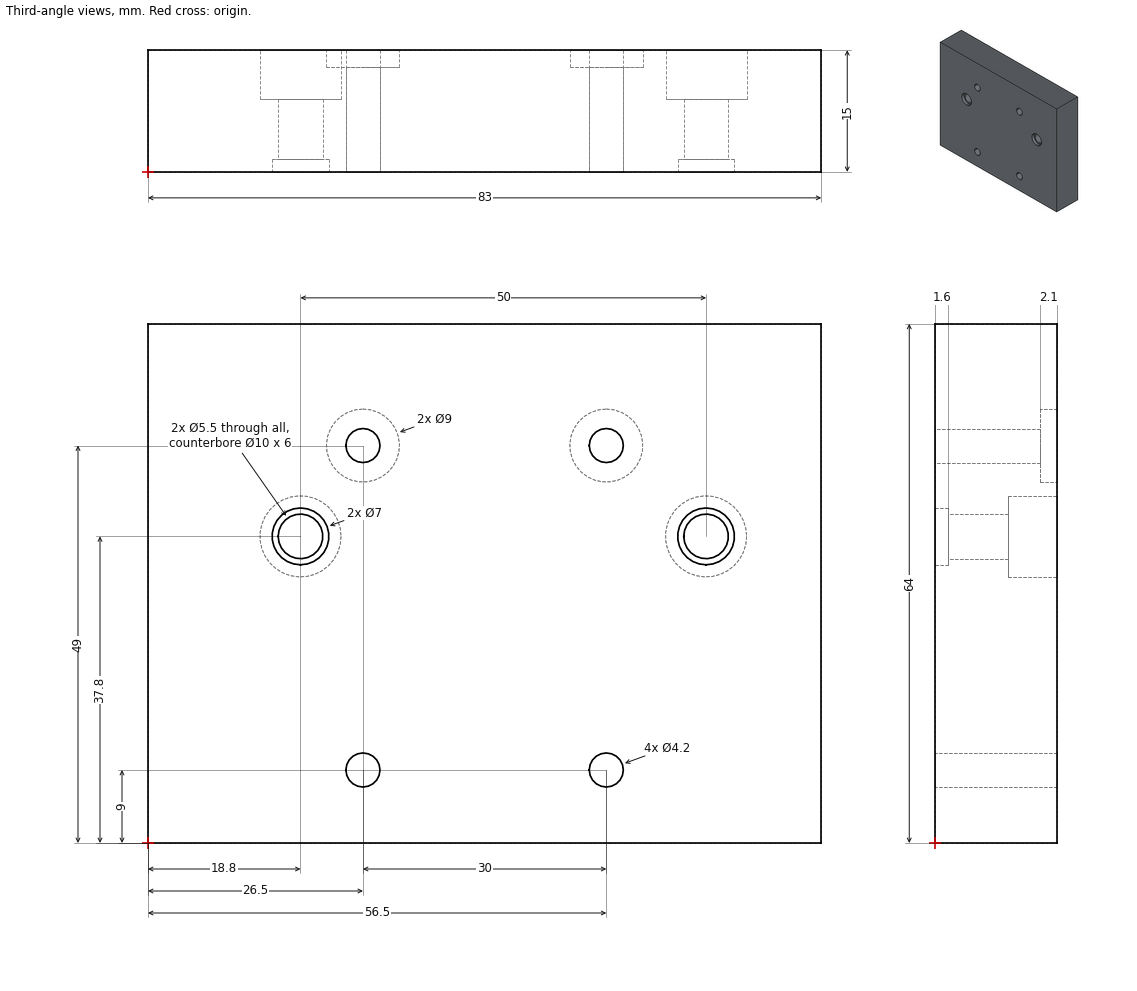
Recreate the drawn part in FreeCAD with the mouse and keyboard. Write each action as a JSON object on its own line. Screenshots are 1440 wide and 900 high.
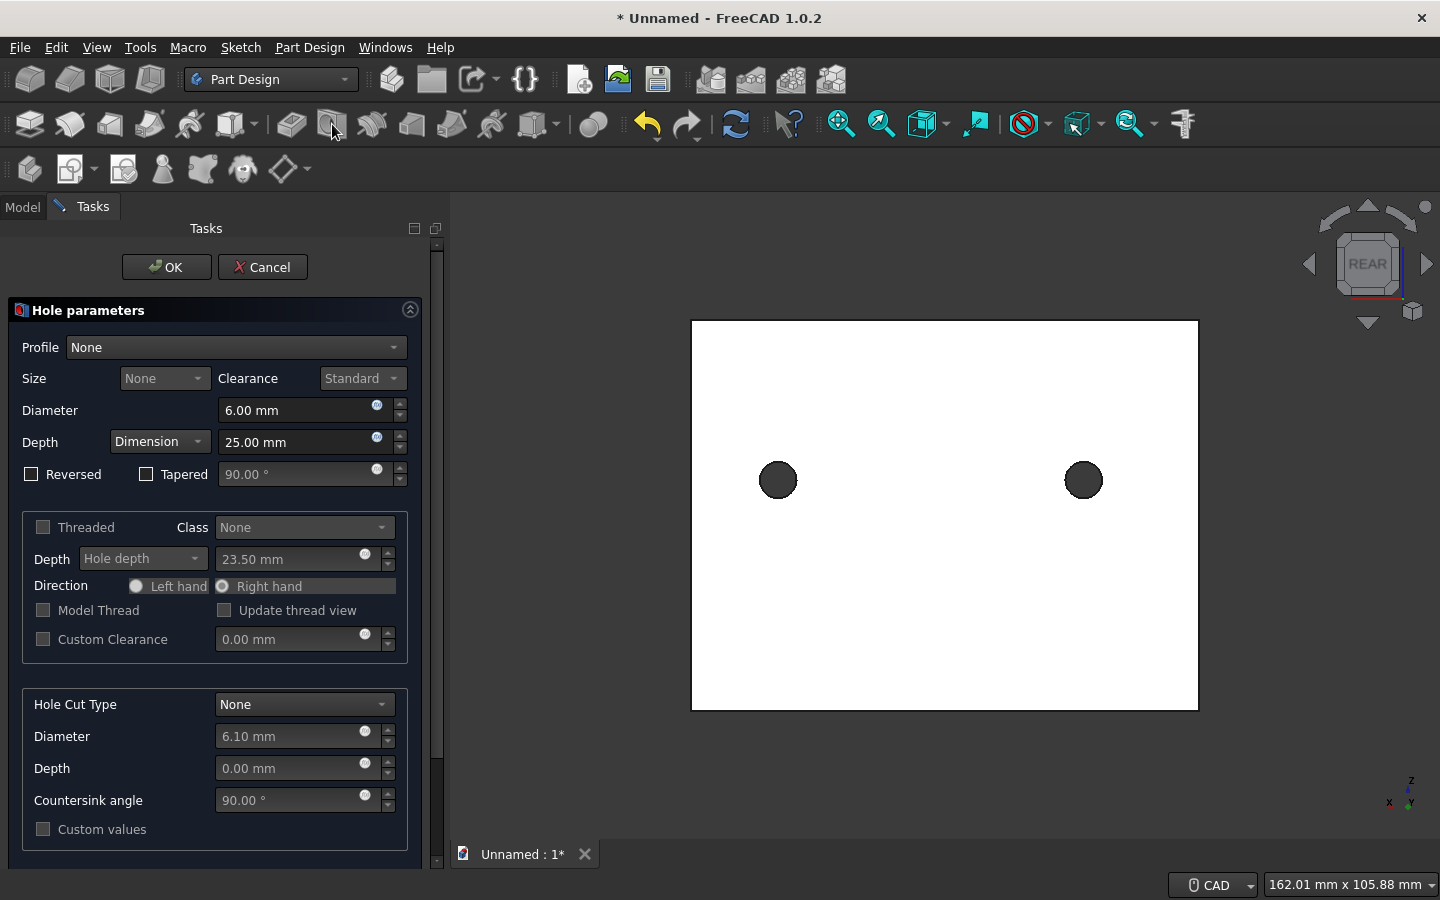
{"action": "triple_click", "coordinate": [305, 410]}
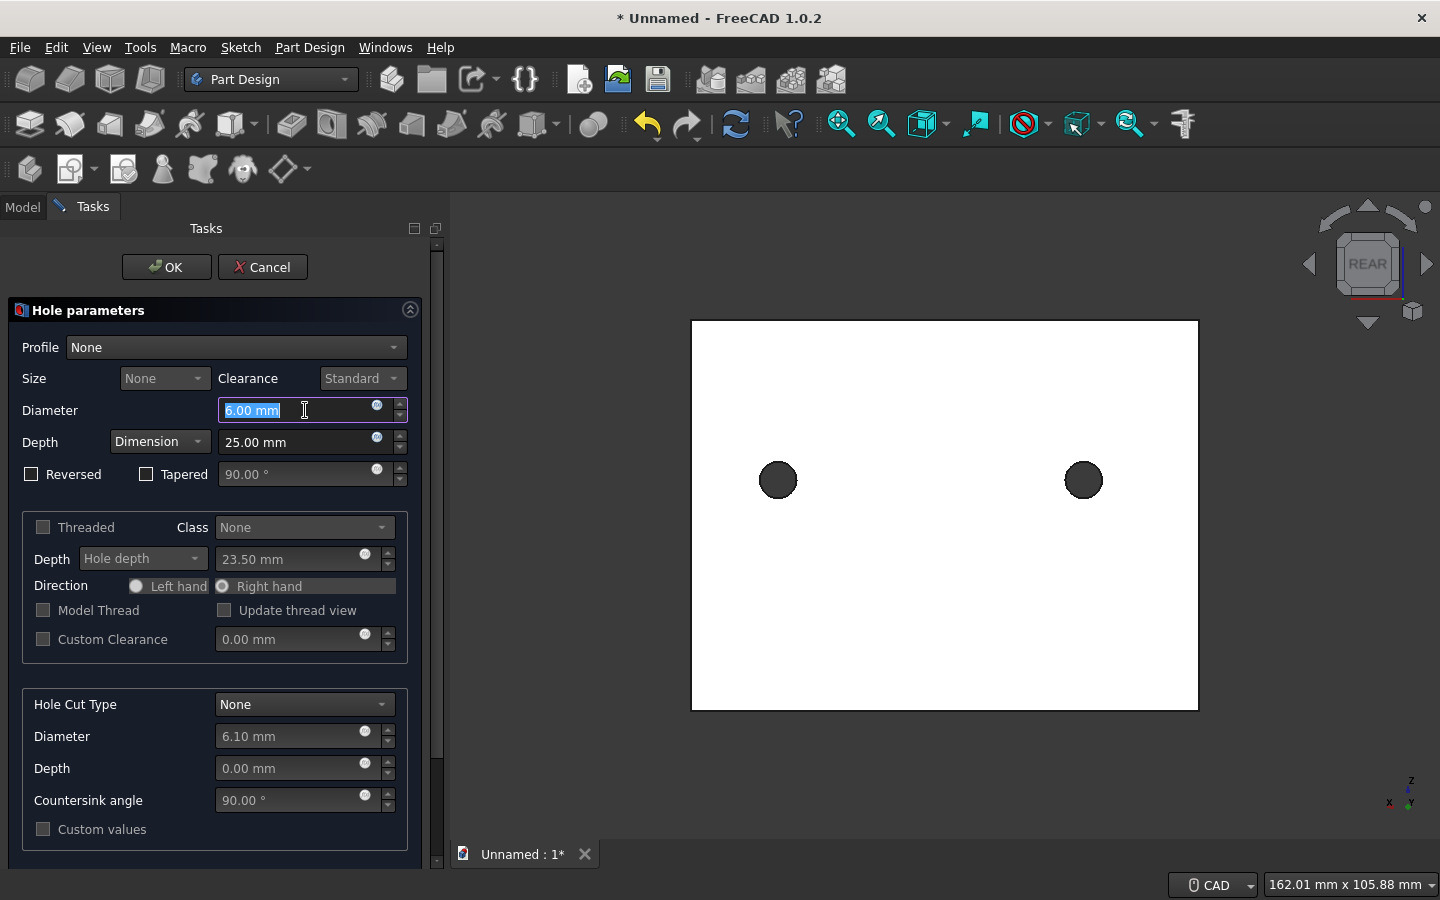
{"action": "type", "text": "5.5"}
{"action": "key", "text": "Tab"}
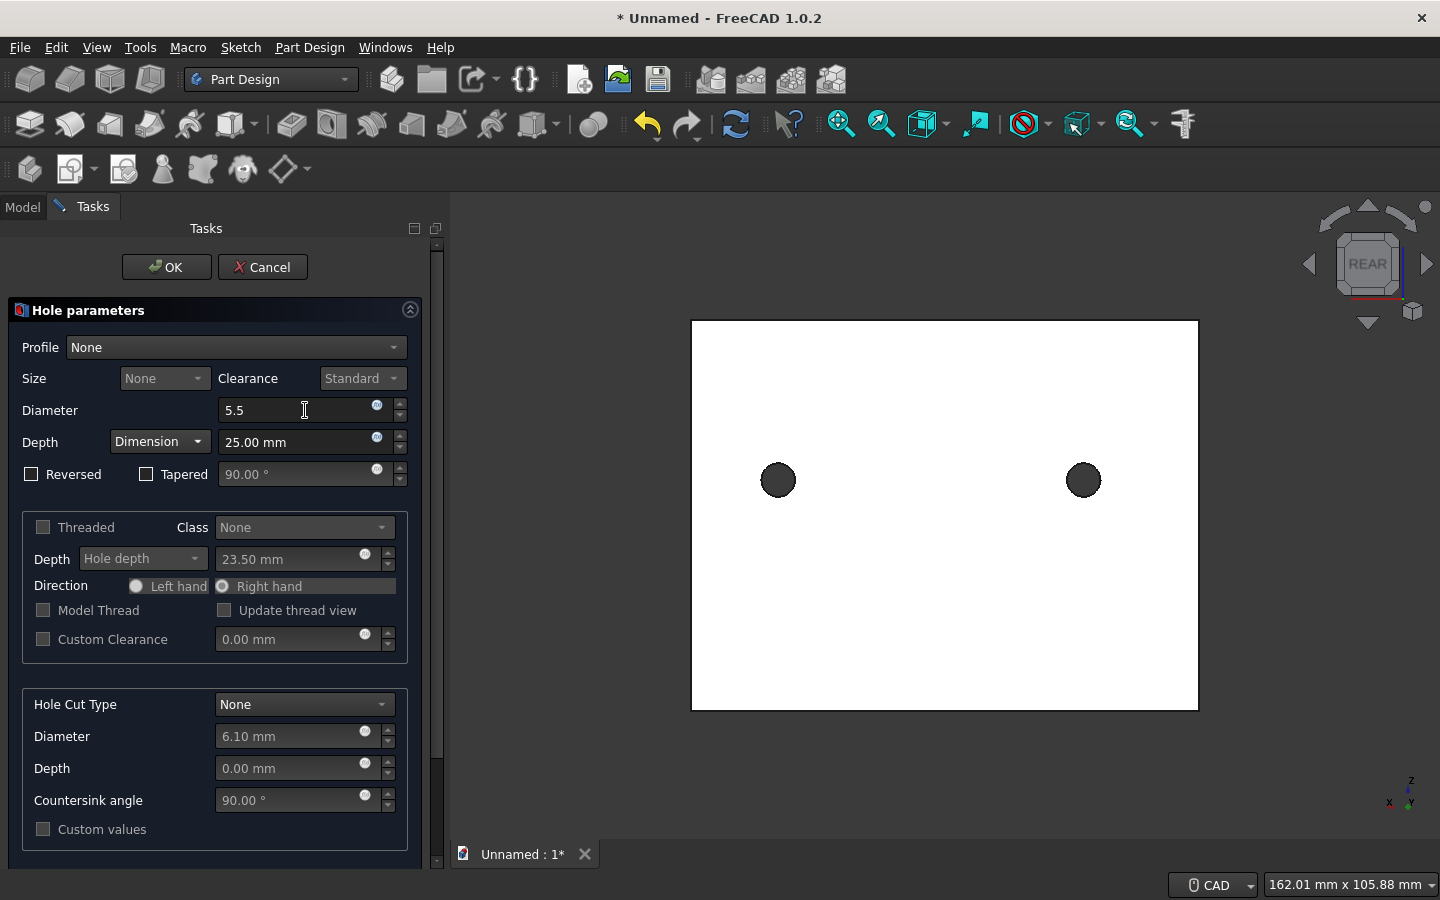
{"action": "left_click", "coordinate": [161, 442]}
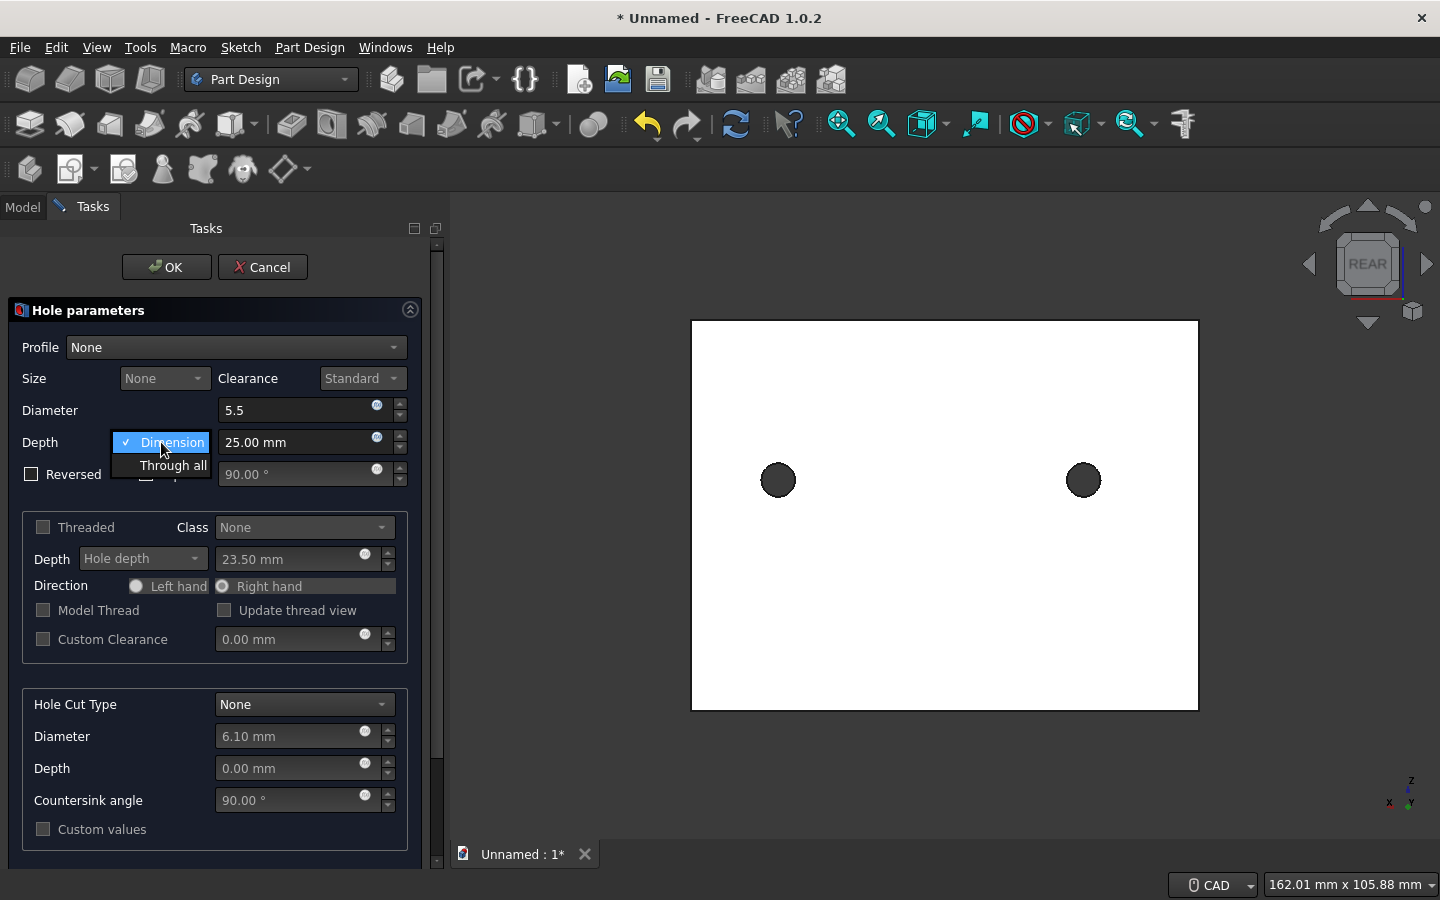
{"action": "left_click", "coordinate": [160, 466]}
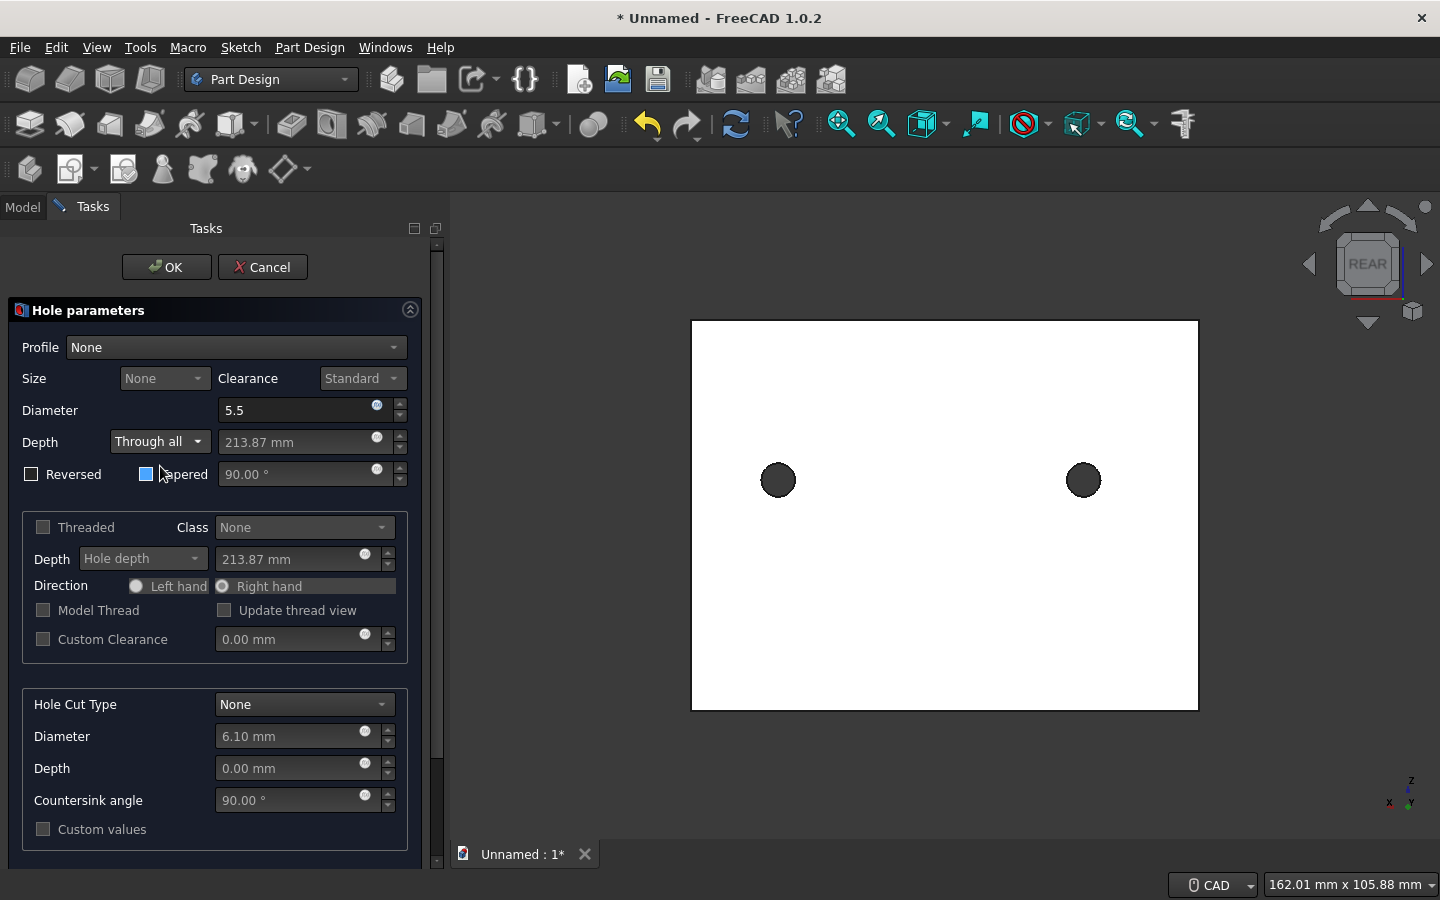
{"action": "left_click", "coordinate": [306, 704]}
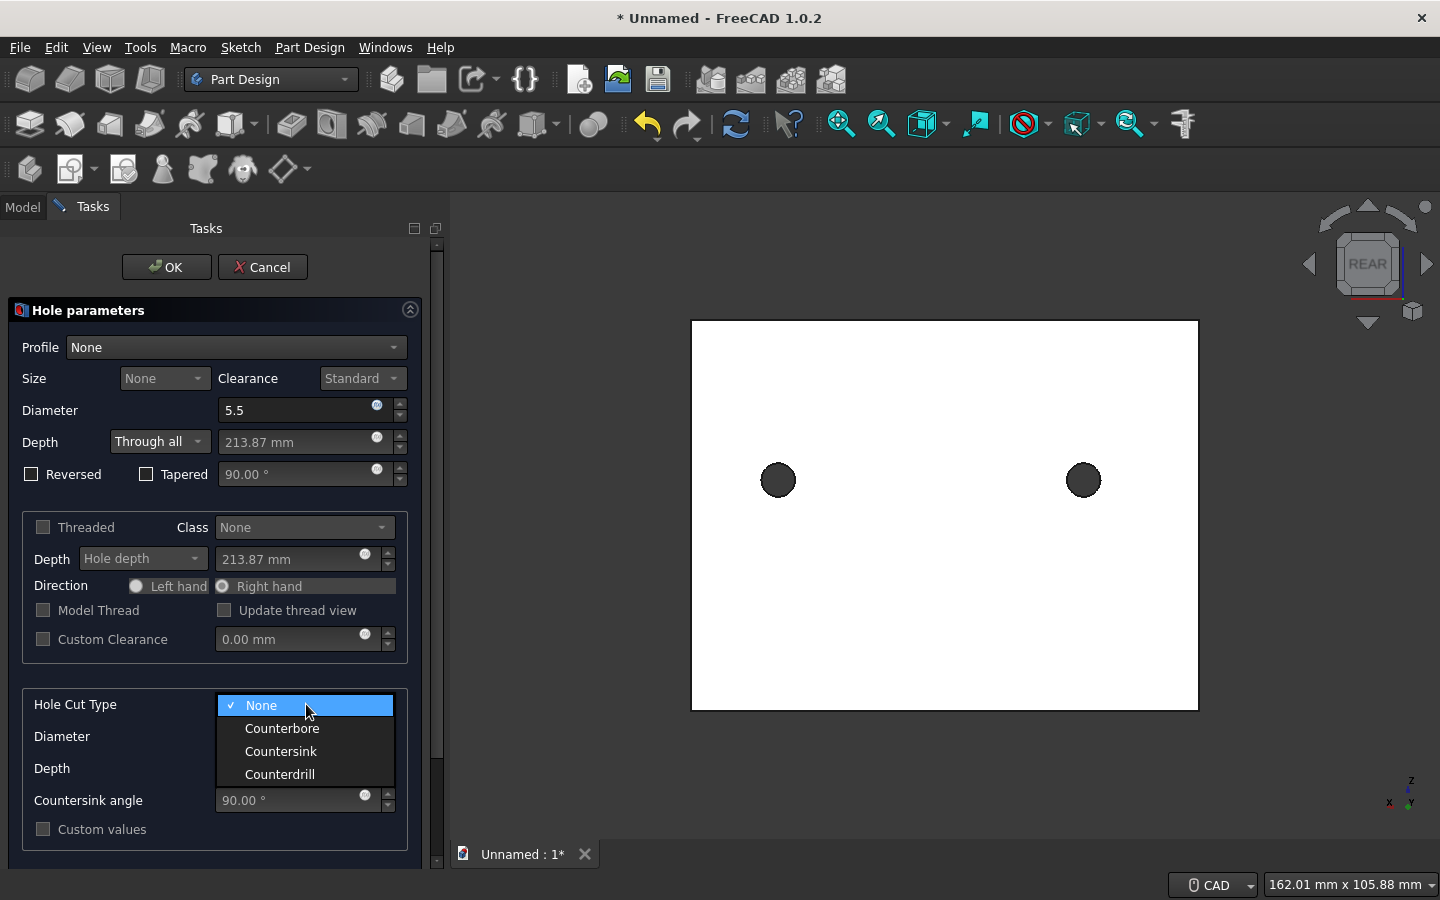
{"action": "left_click", "coordinate": [304, 728]}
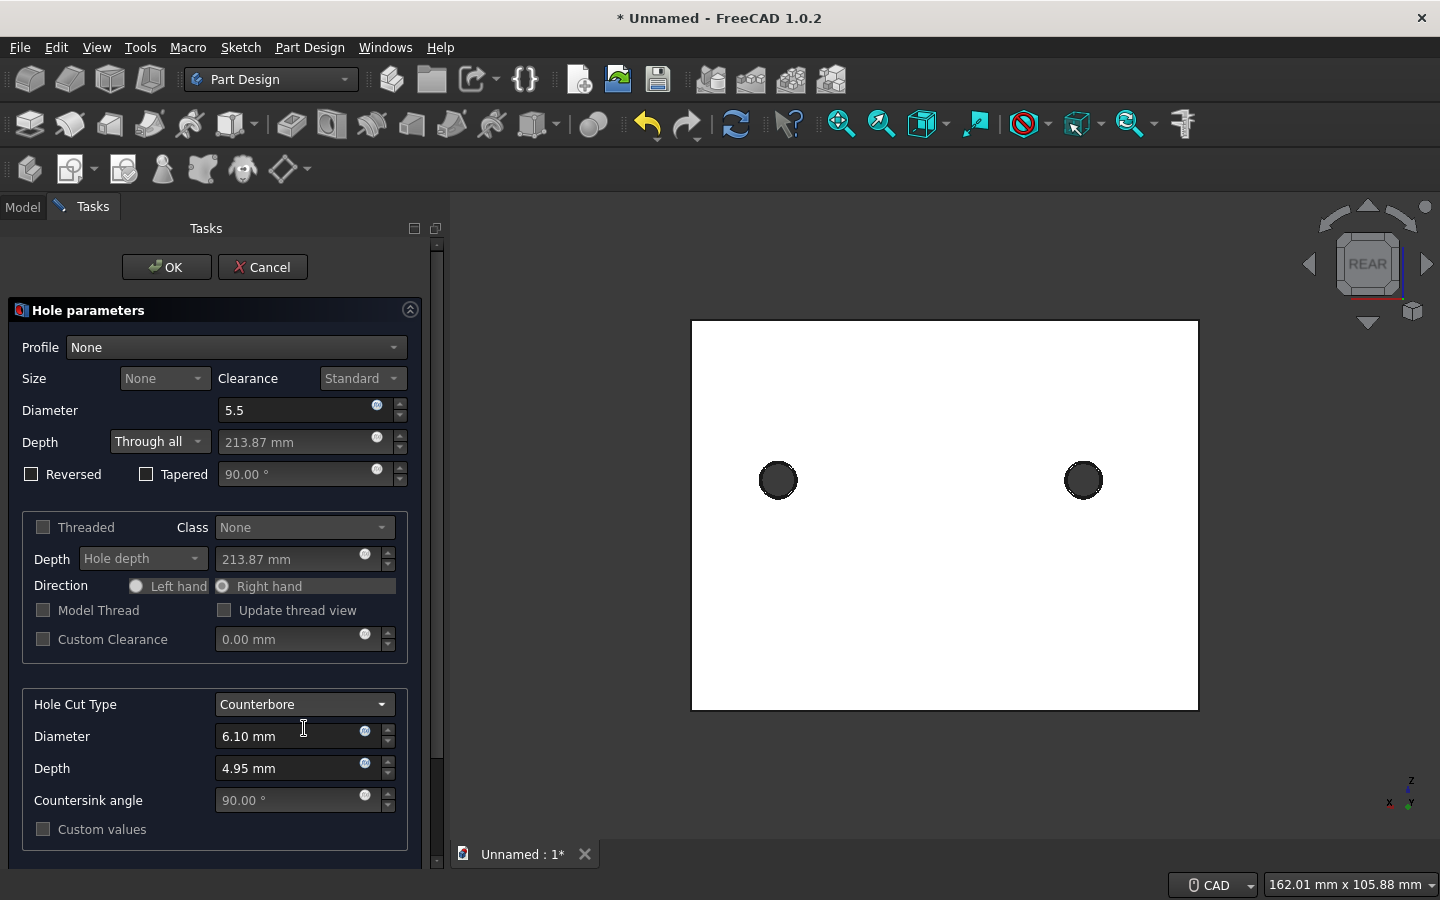
{"action": "triple_click", "coordinate": [298, 736]}